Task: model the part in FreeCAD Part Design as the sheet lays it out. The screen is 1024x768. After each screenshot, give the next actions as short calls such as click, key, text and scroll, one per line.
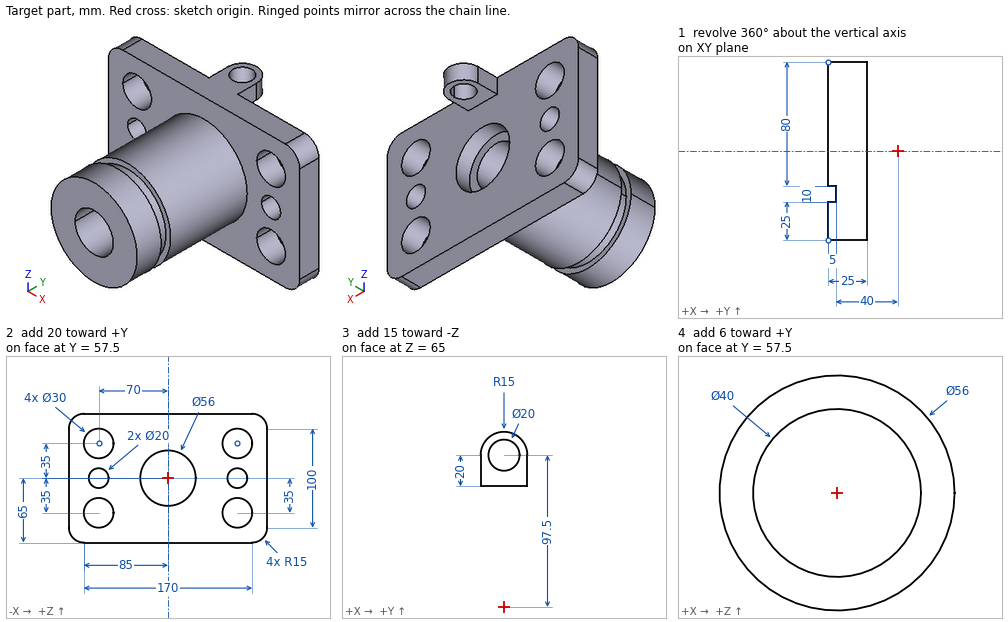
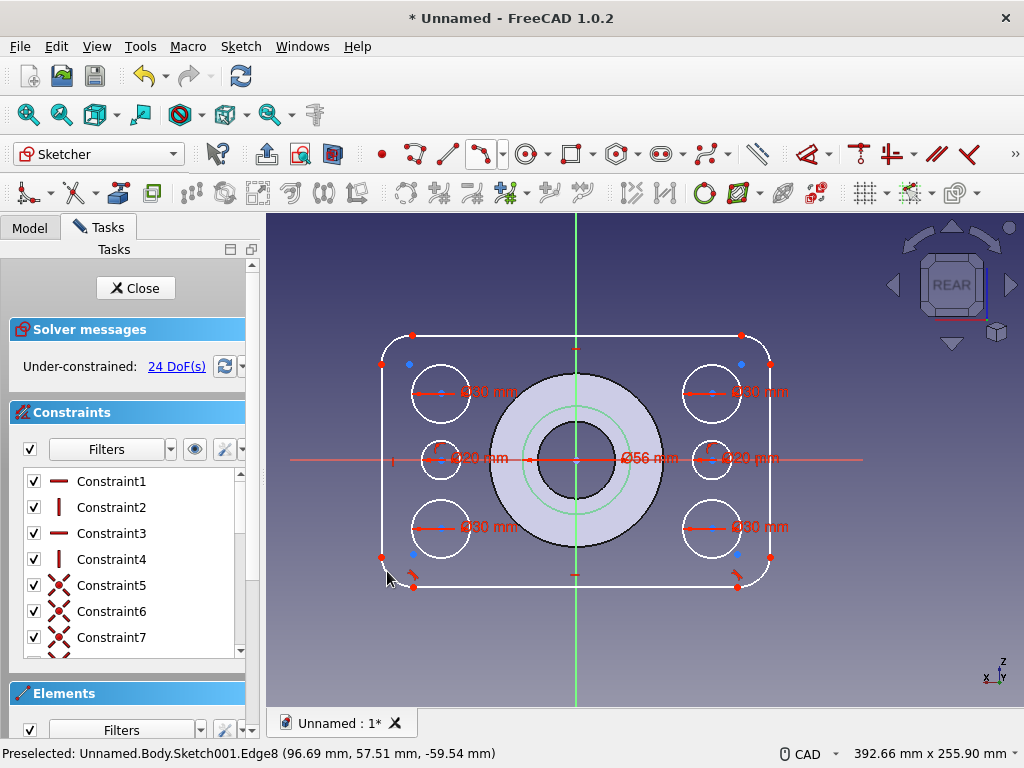
click(770, 500)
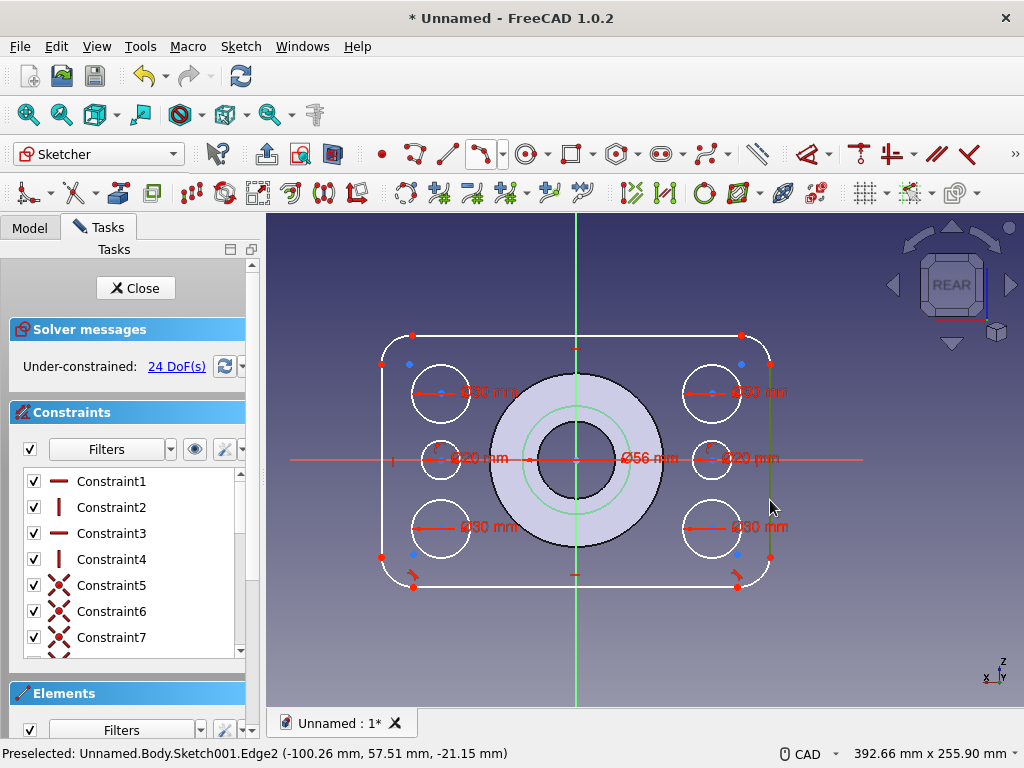
click(752, 584)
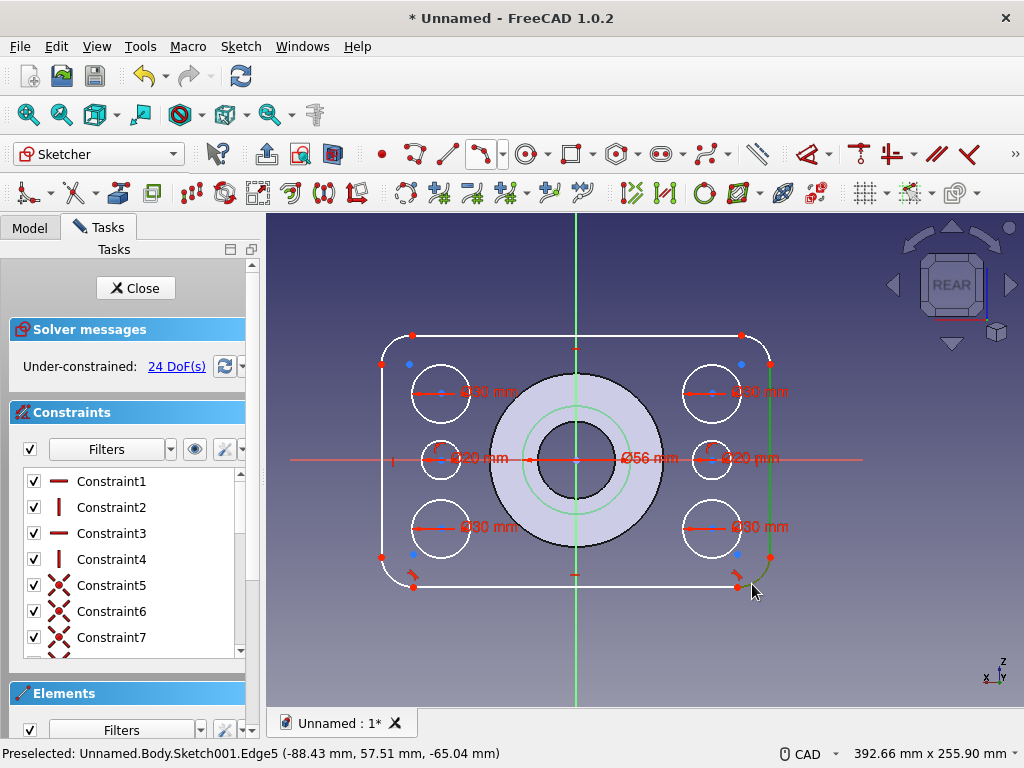
key(t)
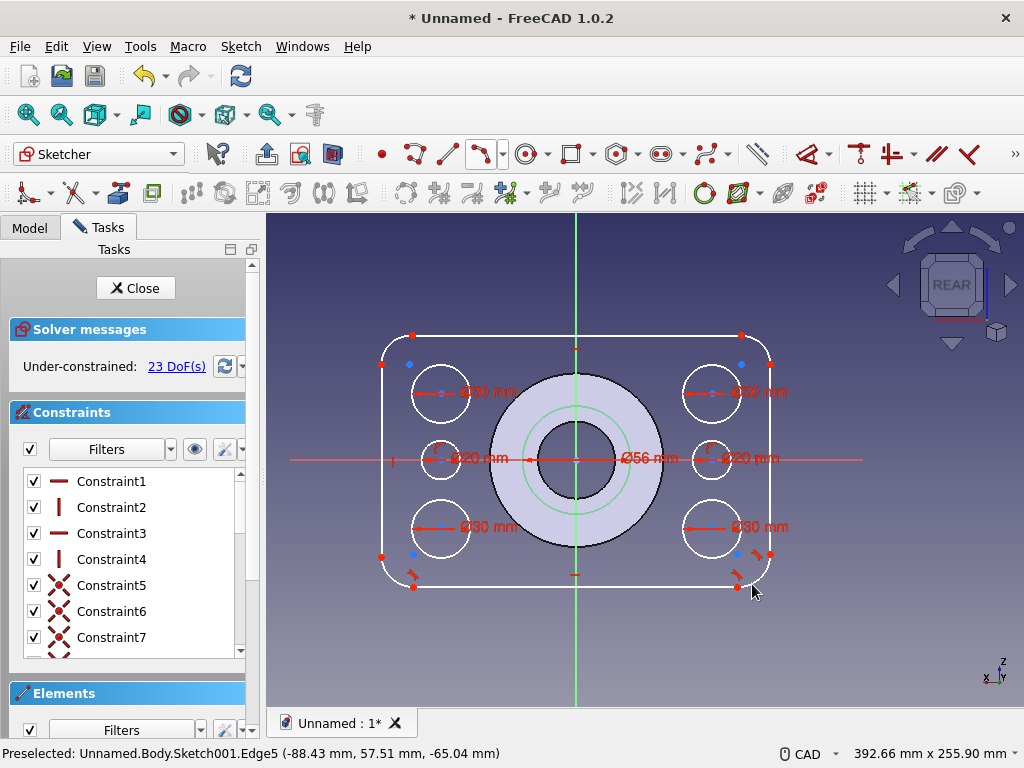
click(770, 498)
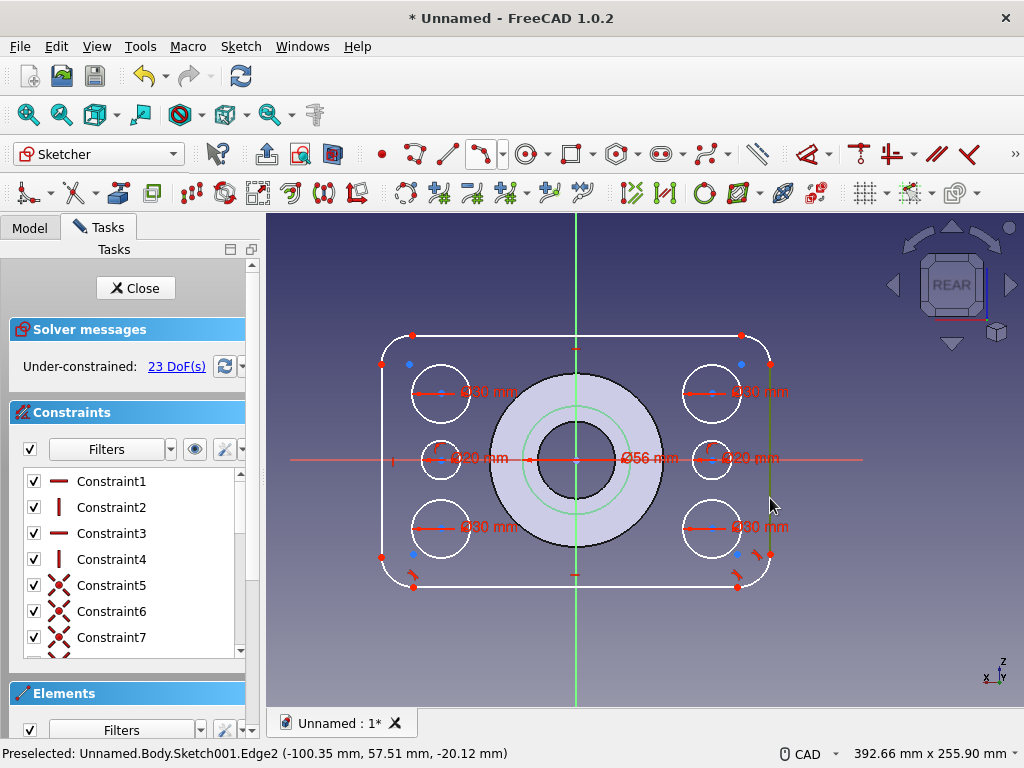
click(767, 352)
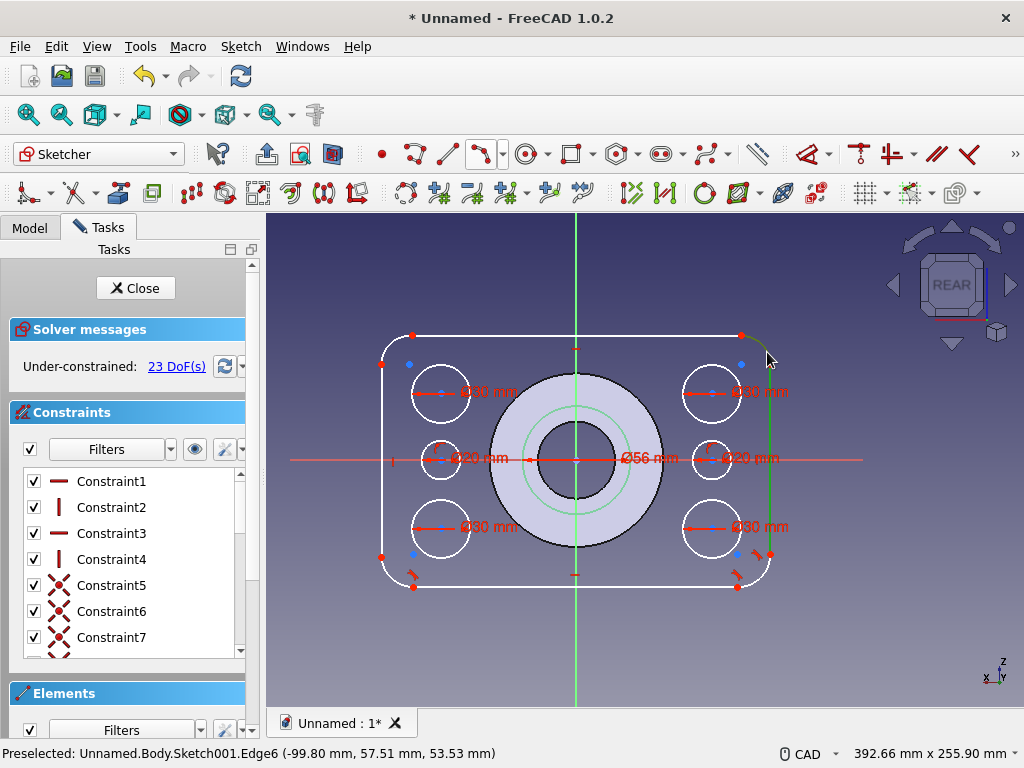
key(t)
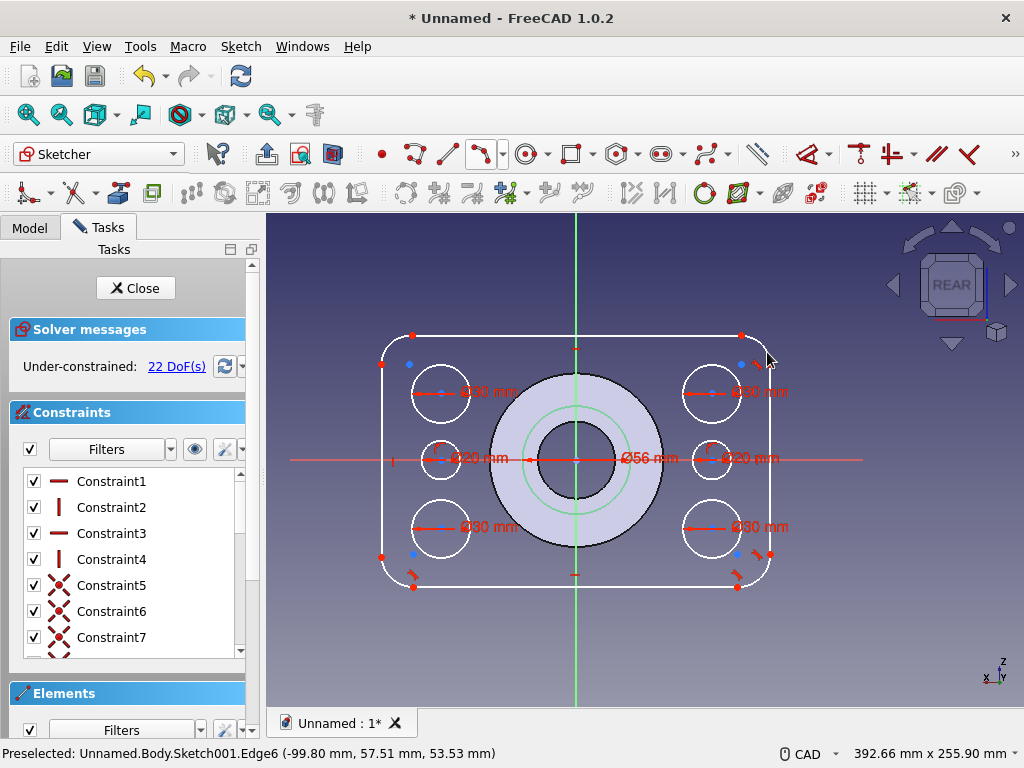
click(642, 336)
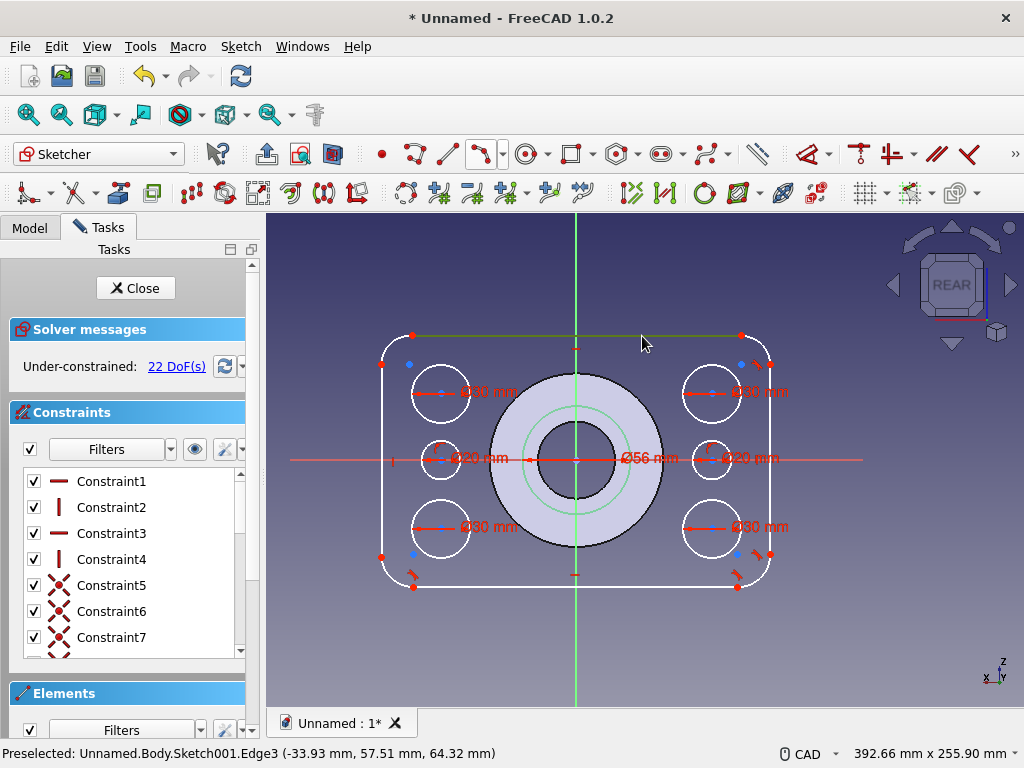
click(767, 352)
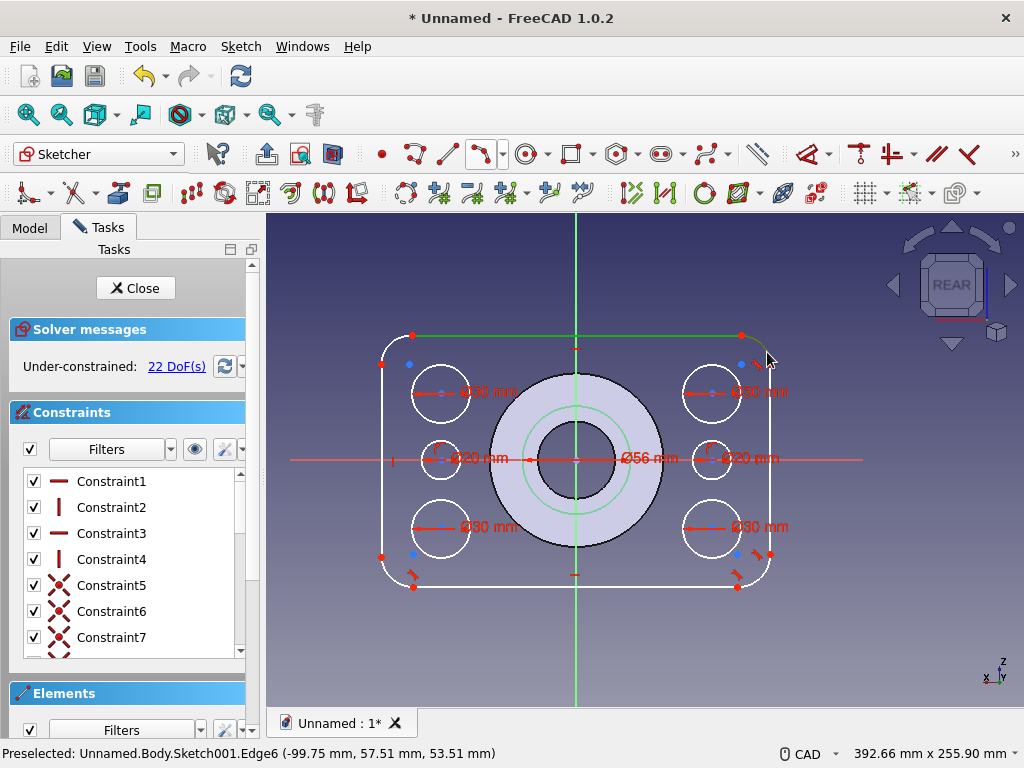
key(t)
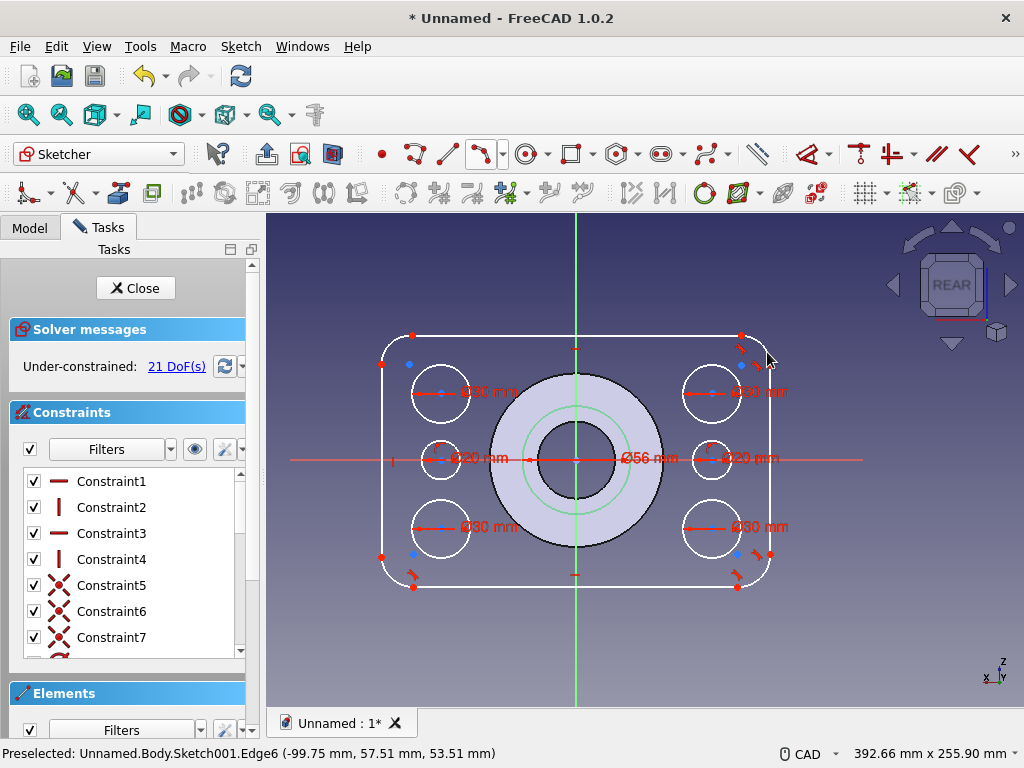
click(642, 336)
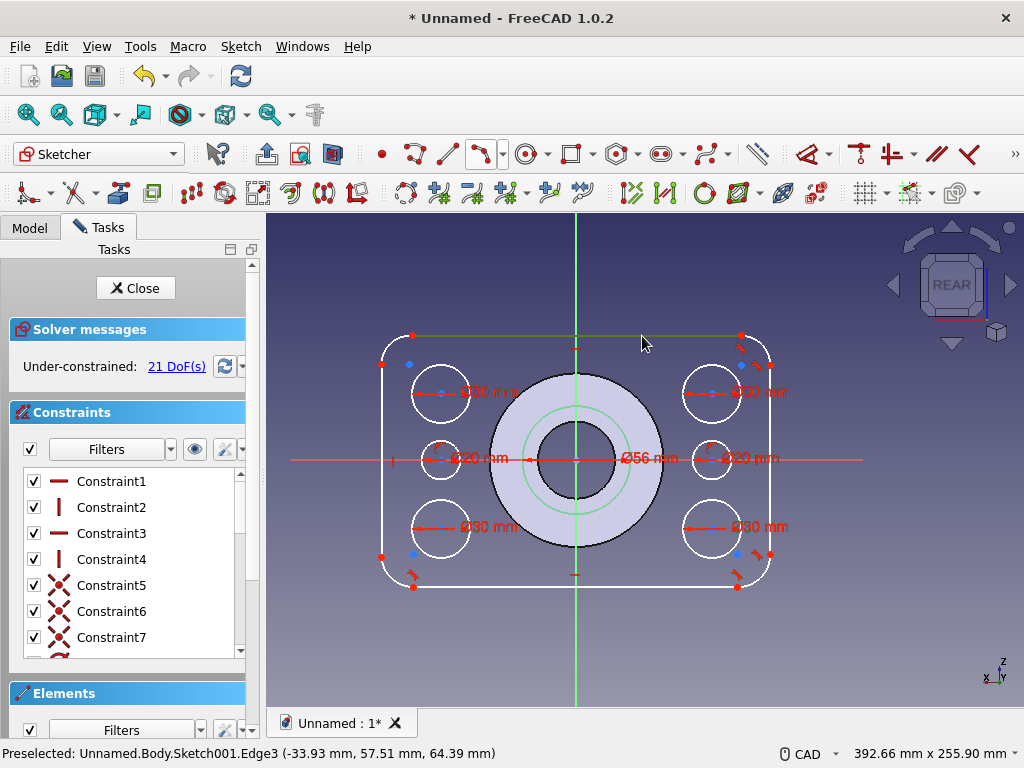
click(398, 338)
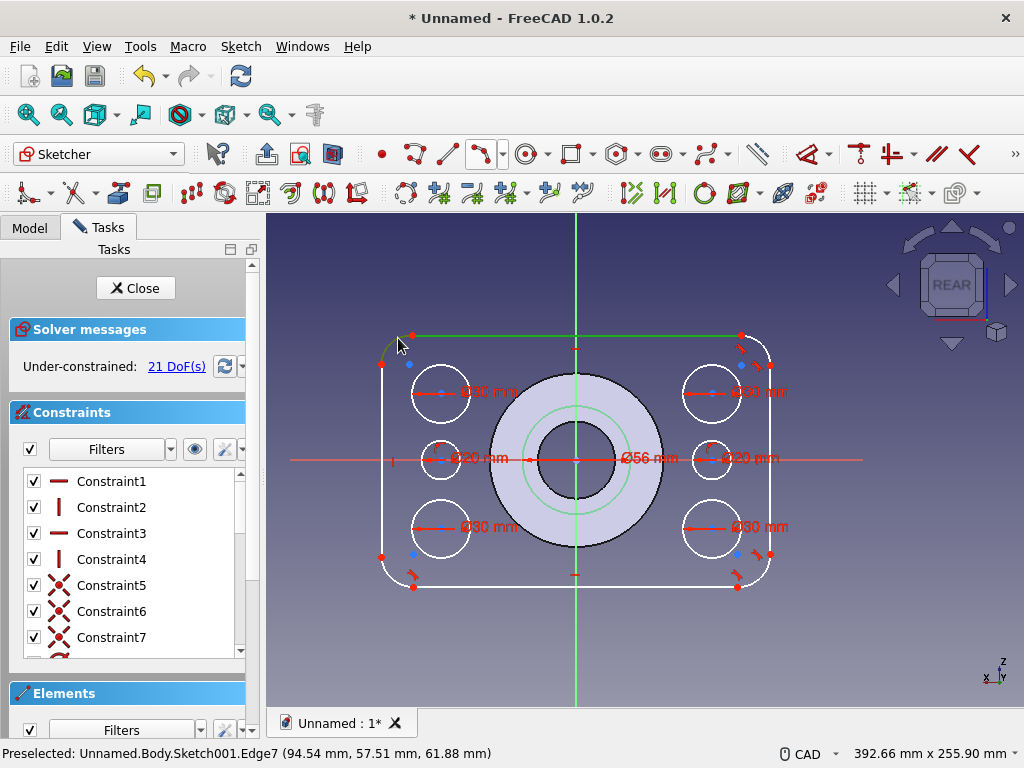
key(t)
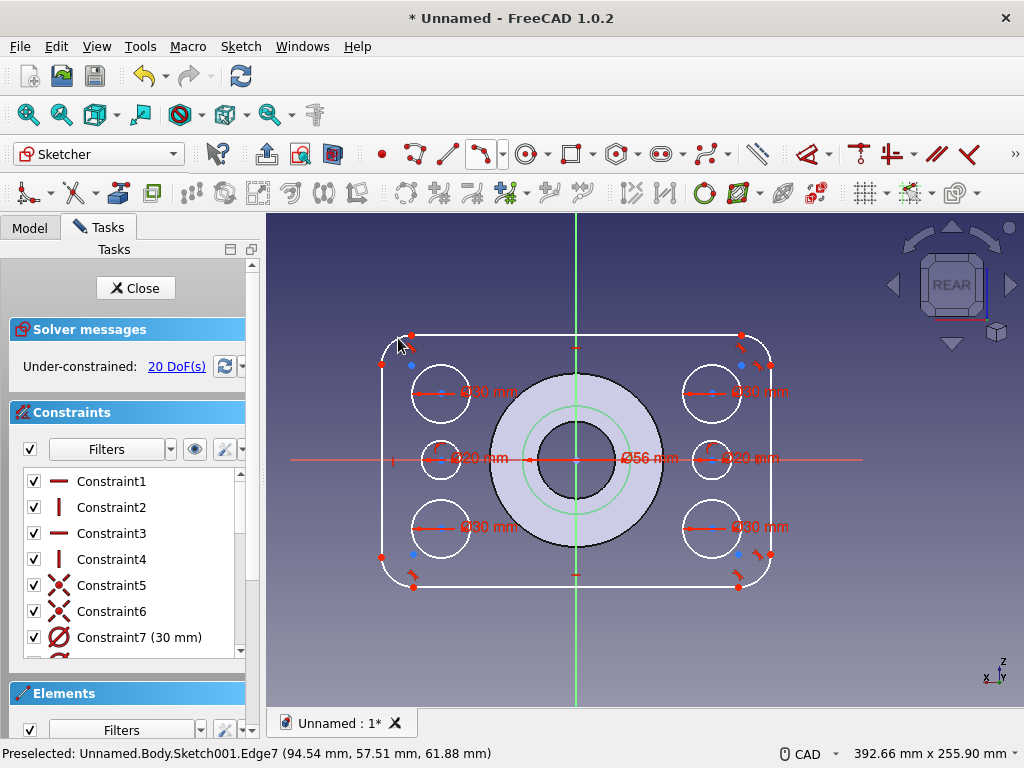
click(382, 423)